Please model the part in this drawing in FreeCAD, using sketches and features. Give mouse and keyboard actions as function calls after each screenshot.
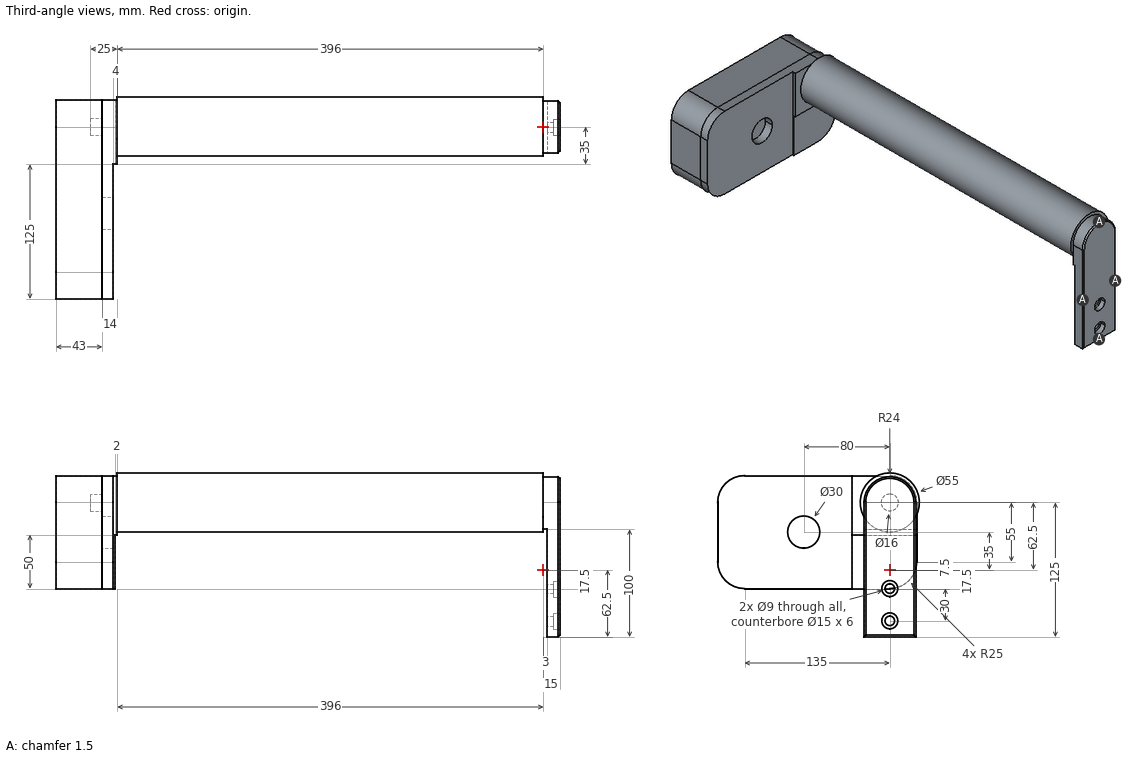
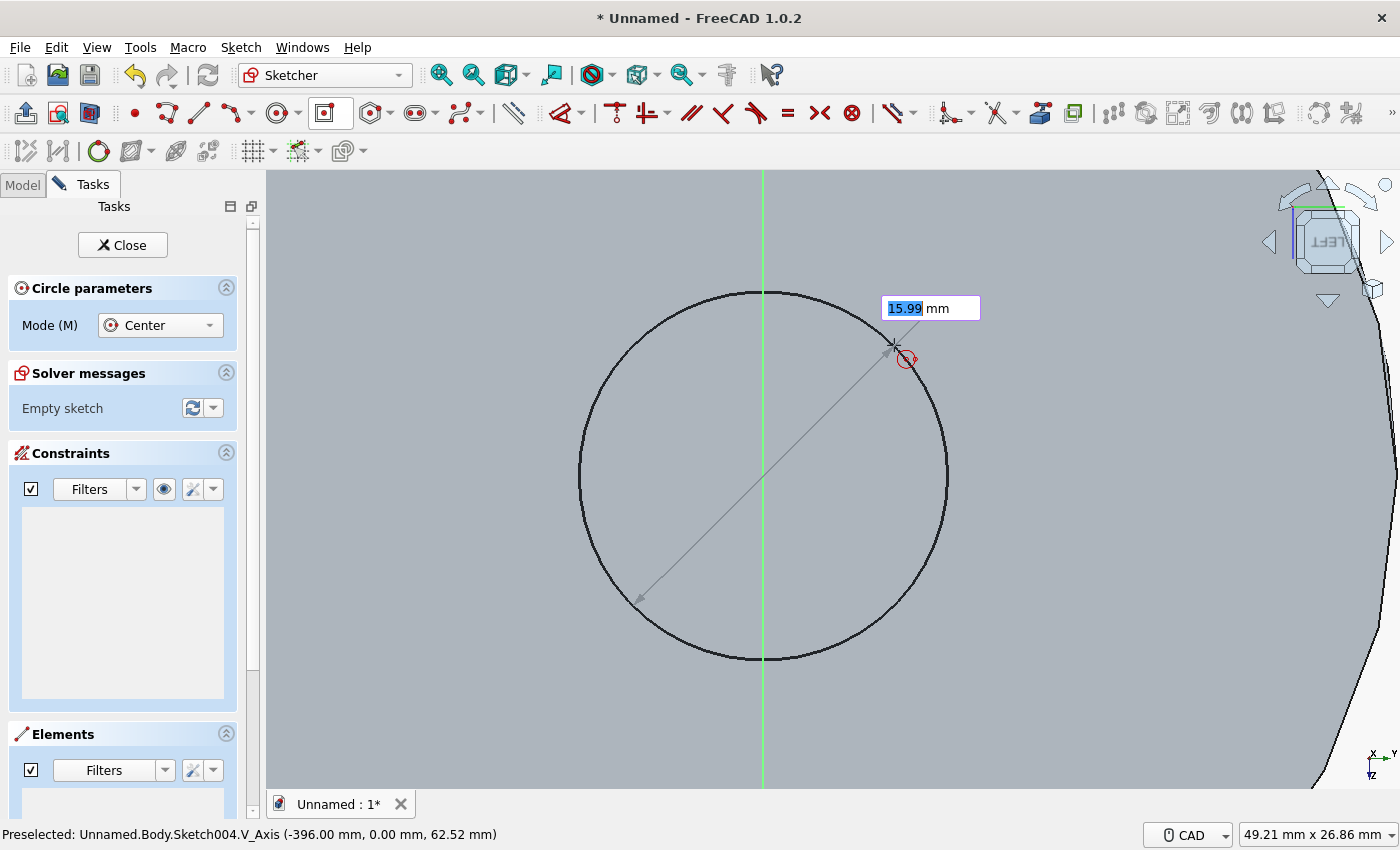
text(16)
key(Return)
key(Escape)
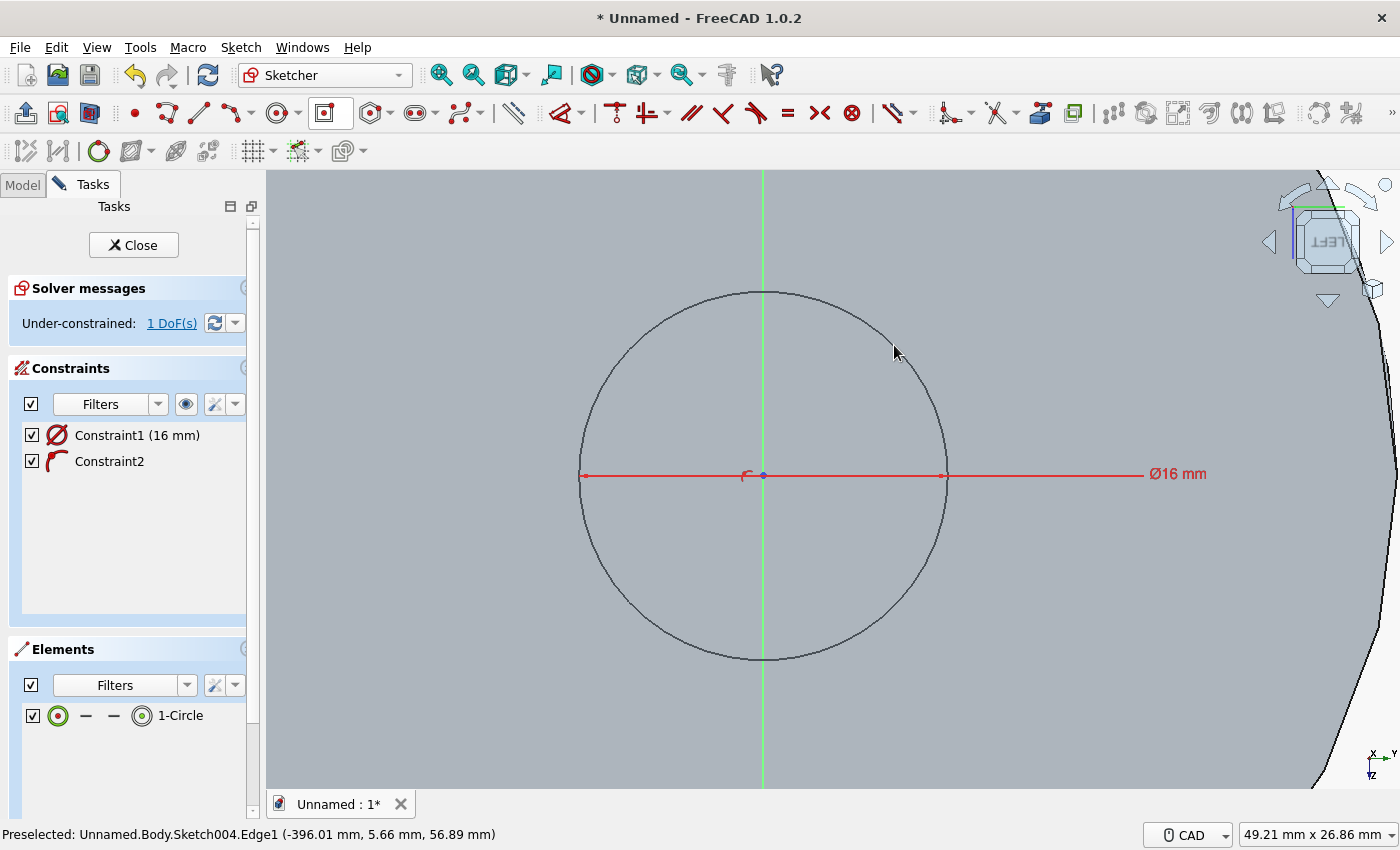
key(d)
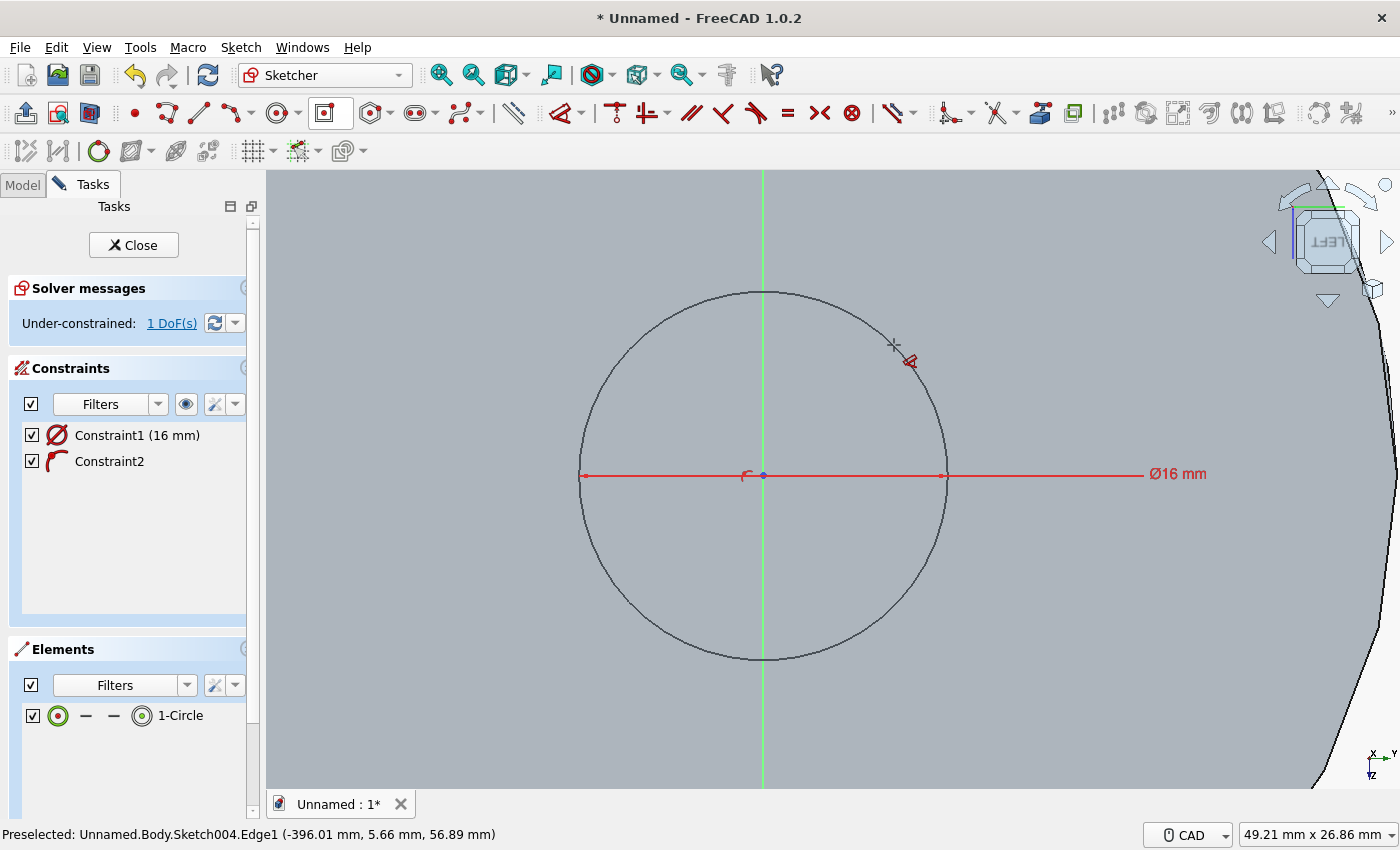
click(763, 476)
click(797, 337)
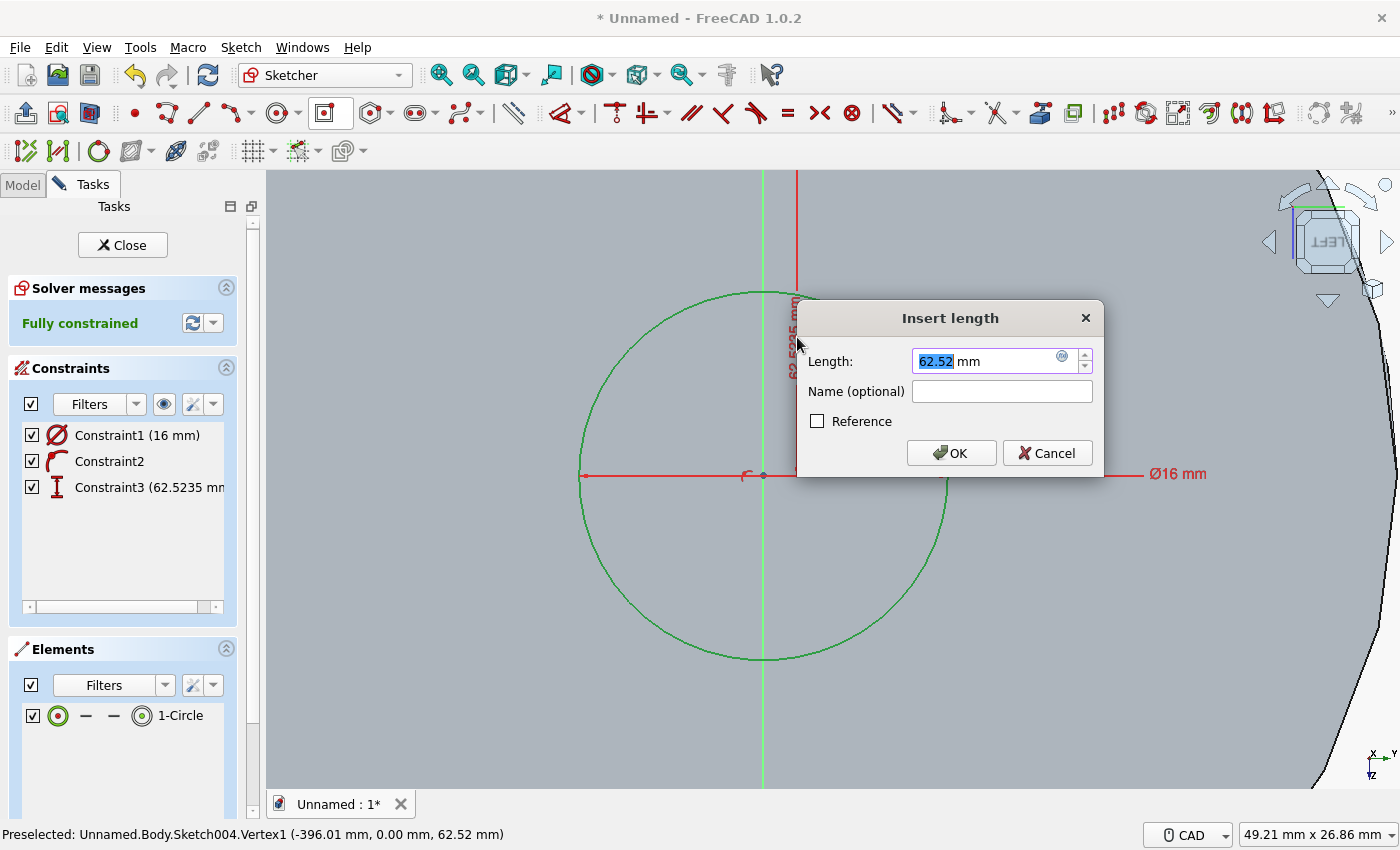
text(62.5)
key(Return)
key(Escape)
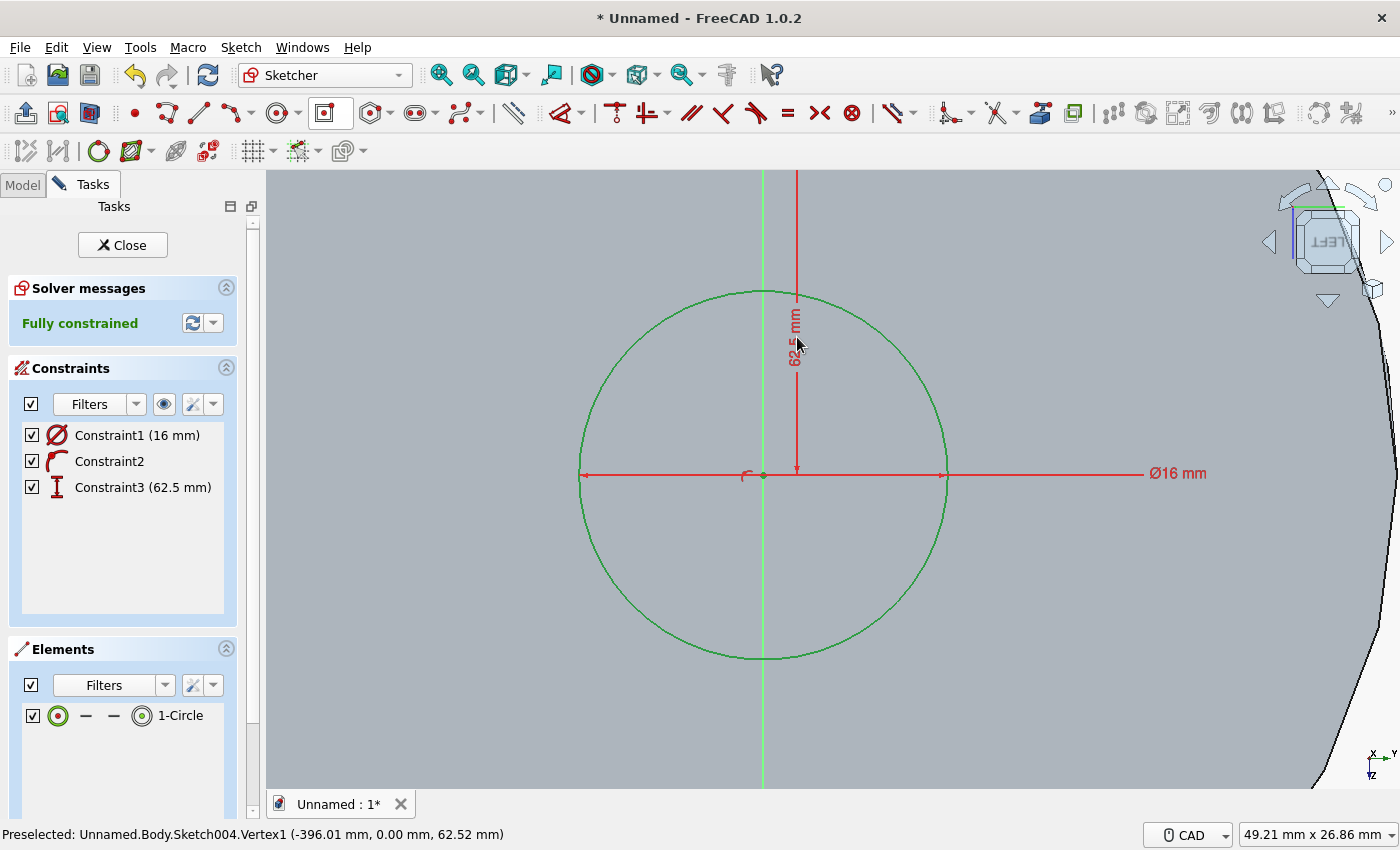
click(123, 245)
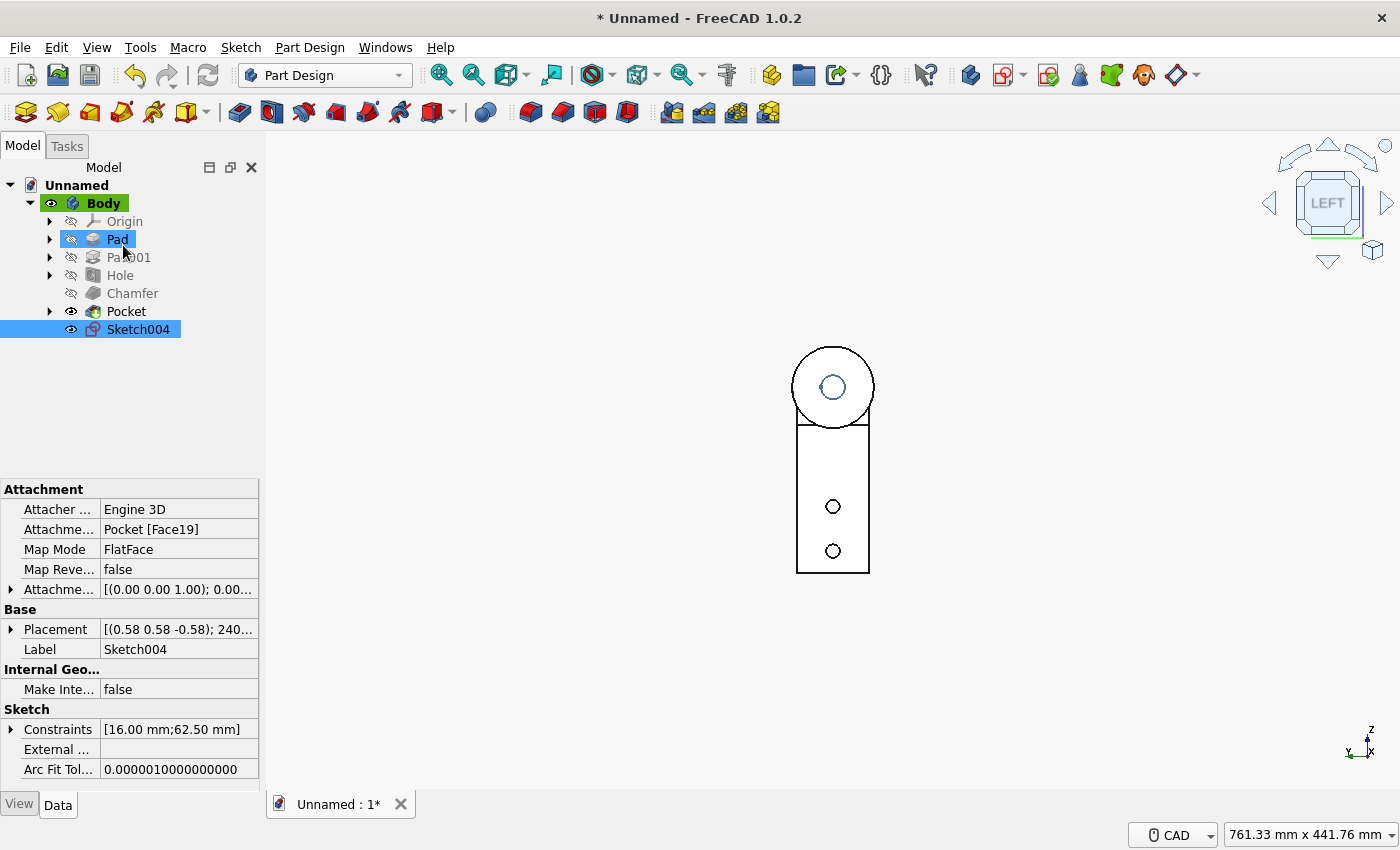
click(26, 112)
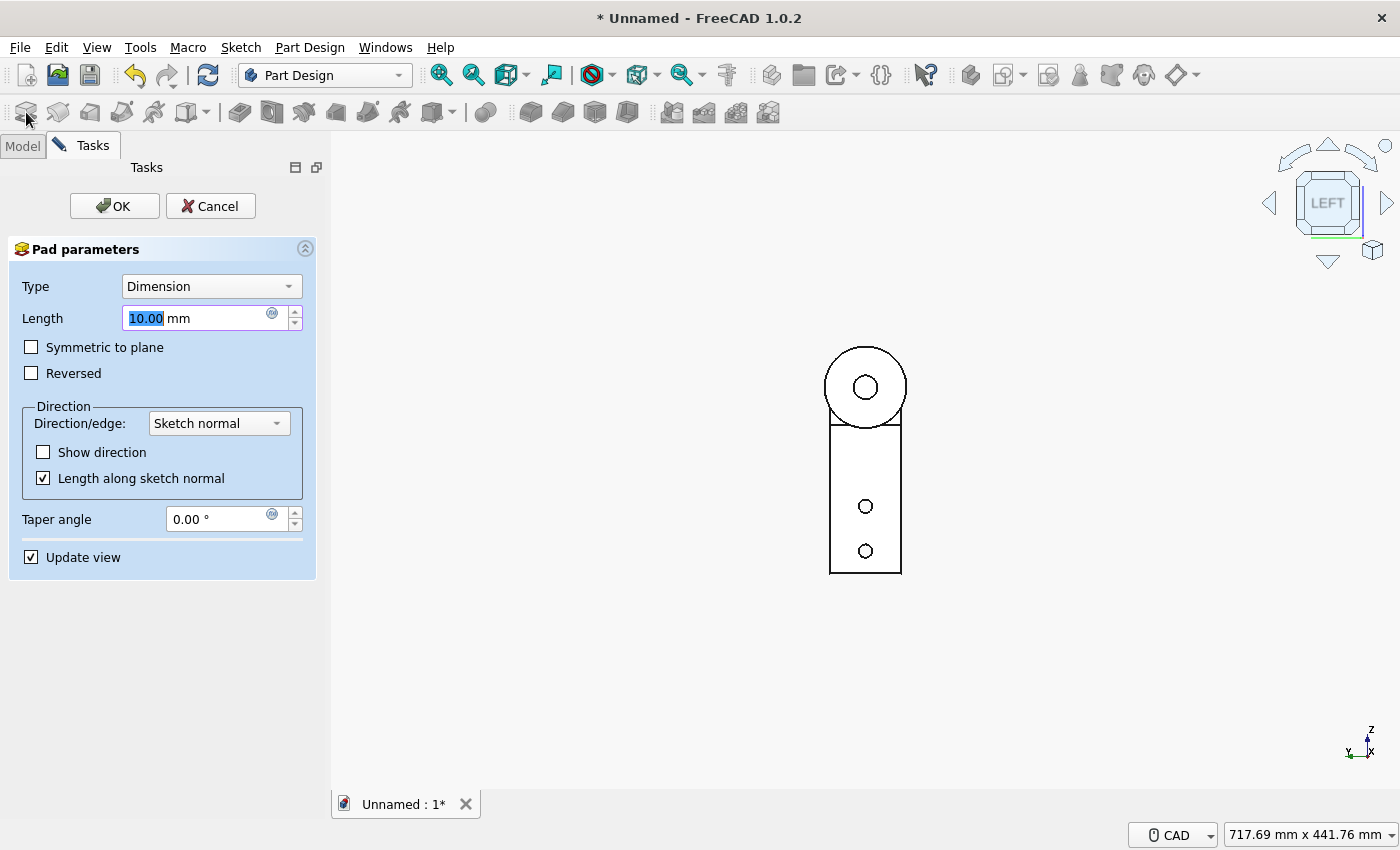
text(25)
key(Tab)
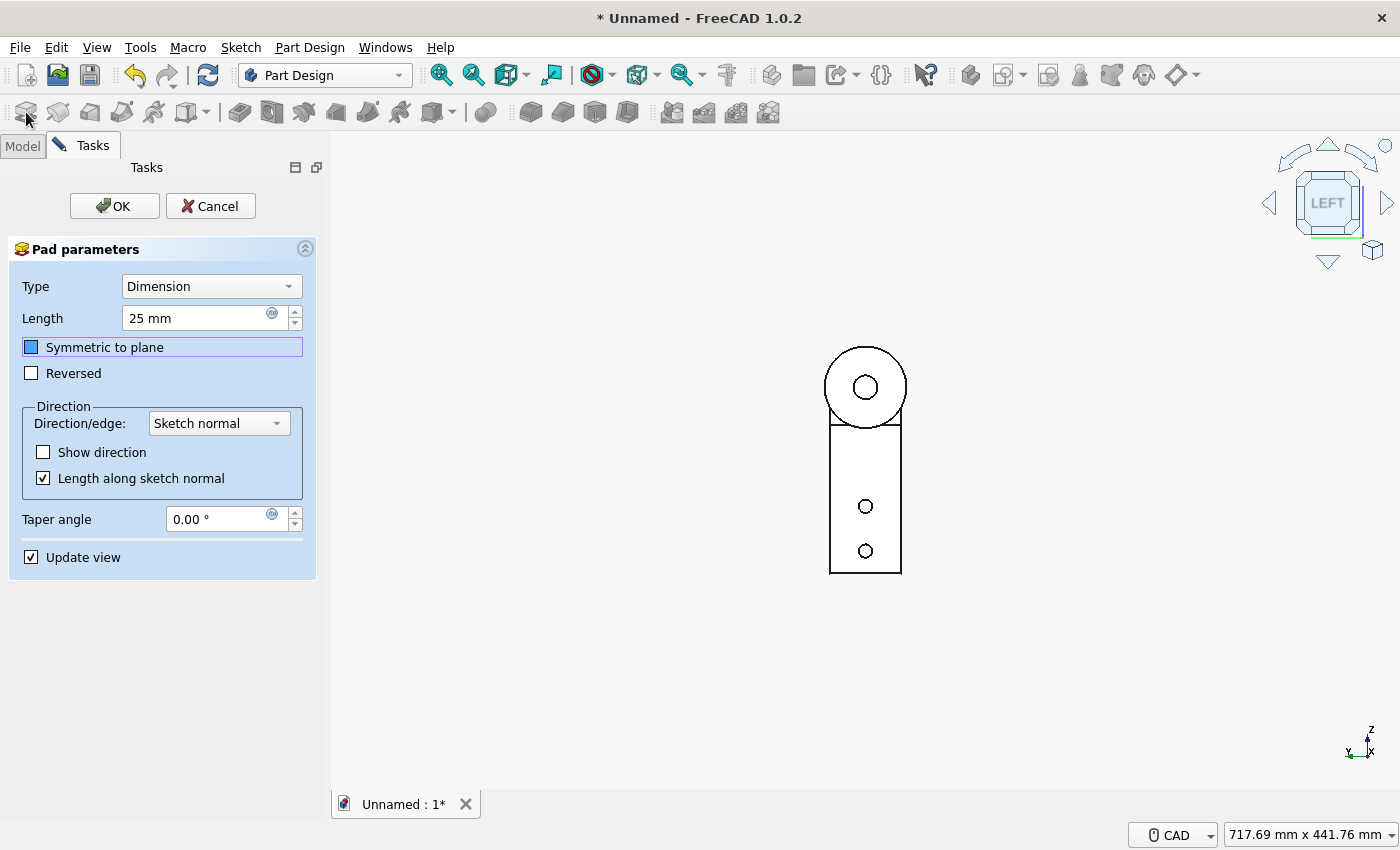
click(115, 206)